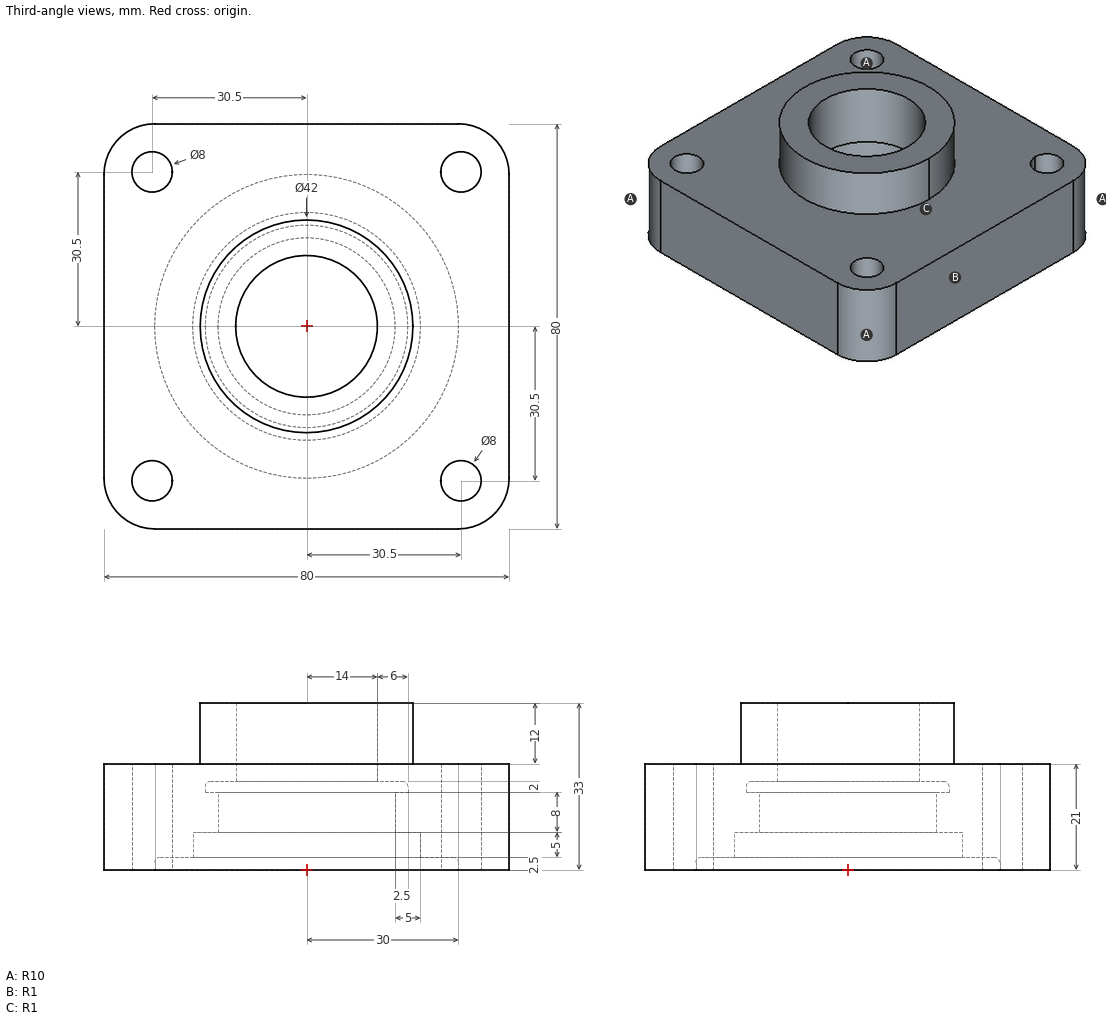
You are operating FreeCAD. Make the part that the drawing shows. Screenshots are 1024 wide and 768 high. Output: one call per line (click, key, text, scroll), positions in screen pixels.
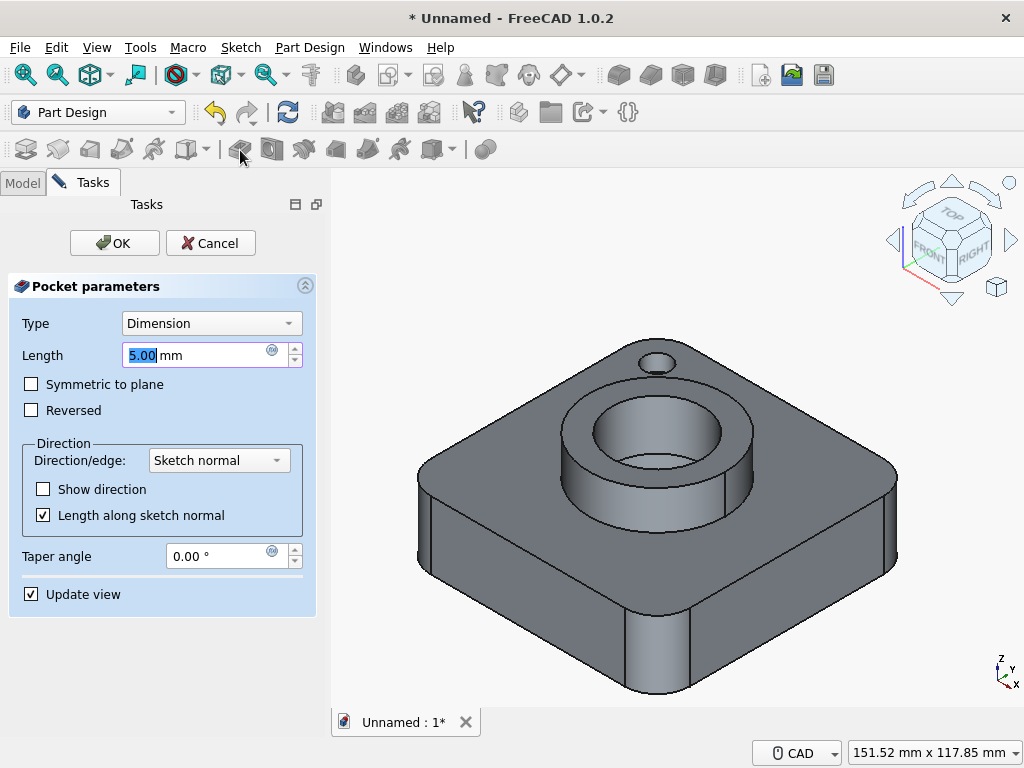
text(21)
key(Tab)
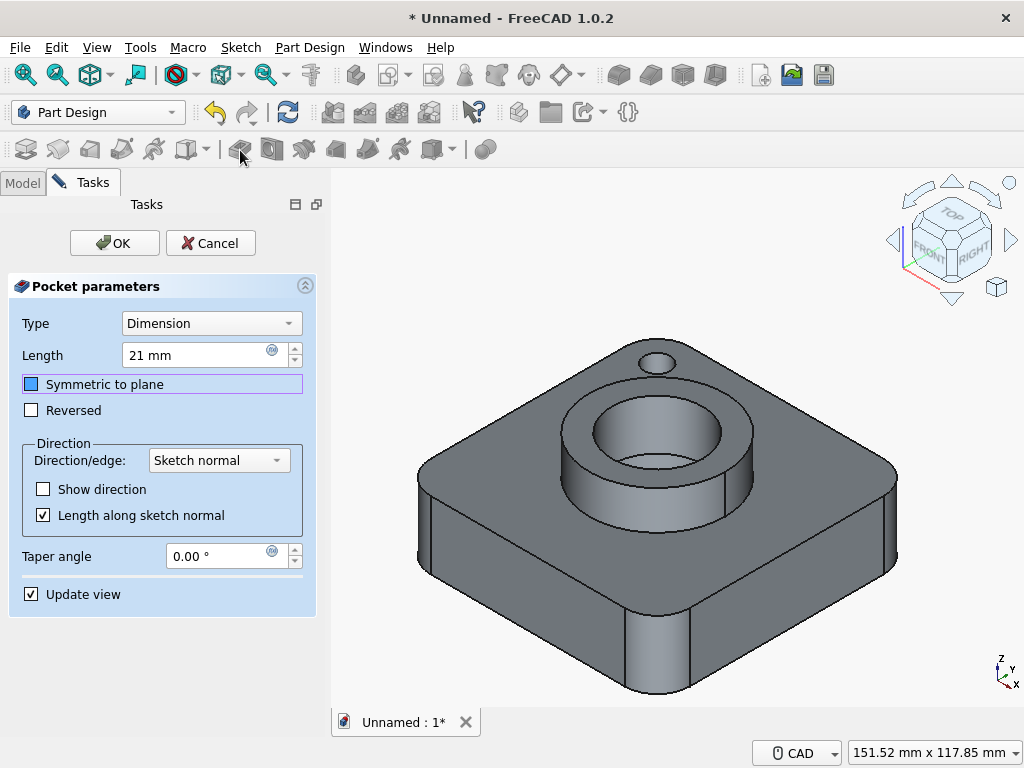
click(115, 243)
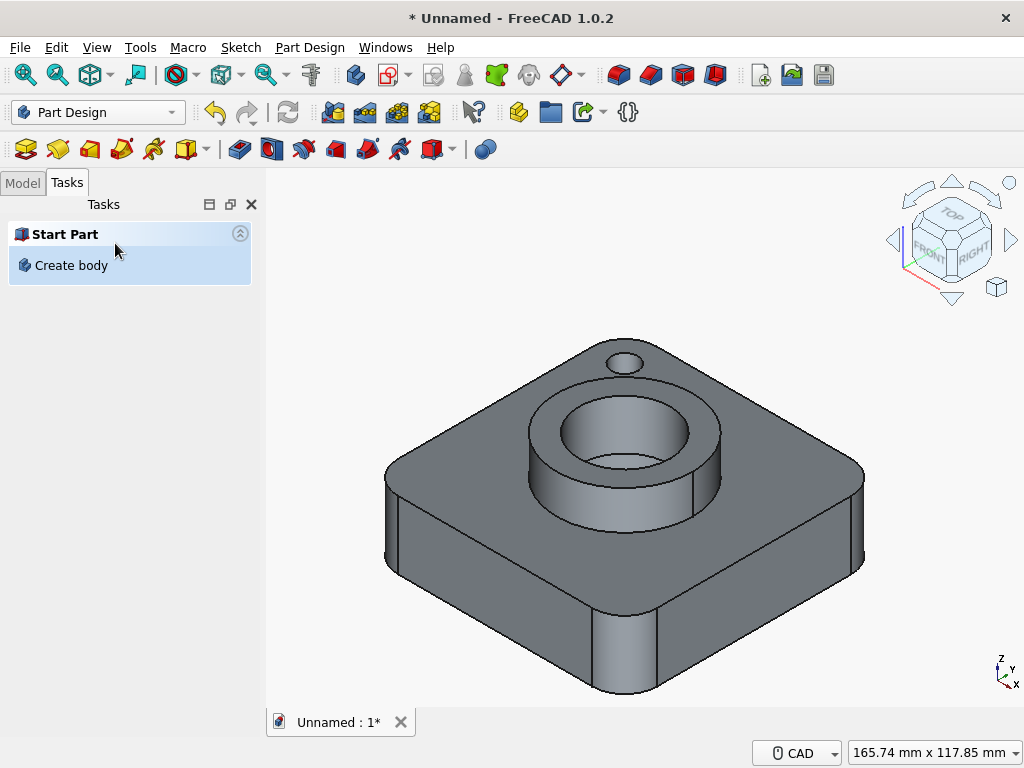
click(23, 182)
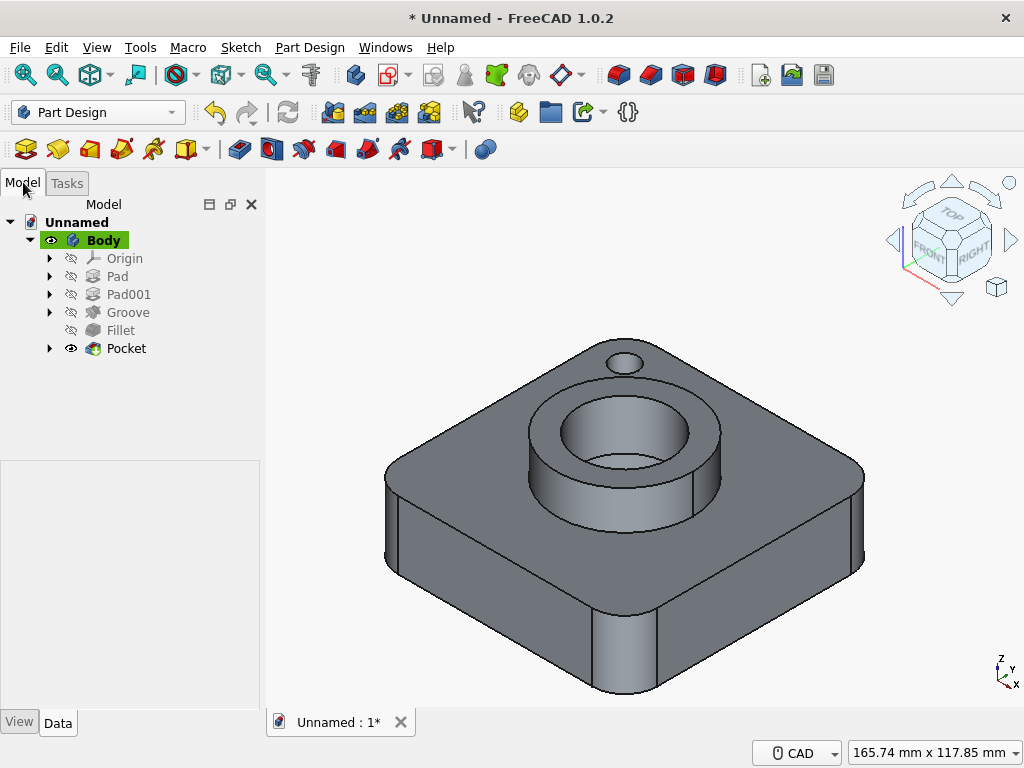
click(116, 348)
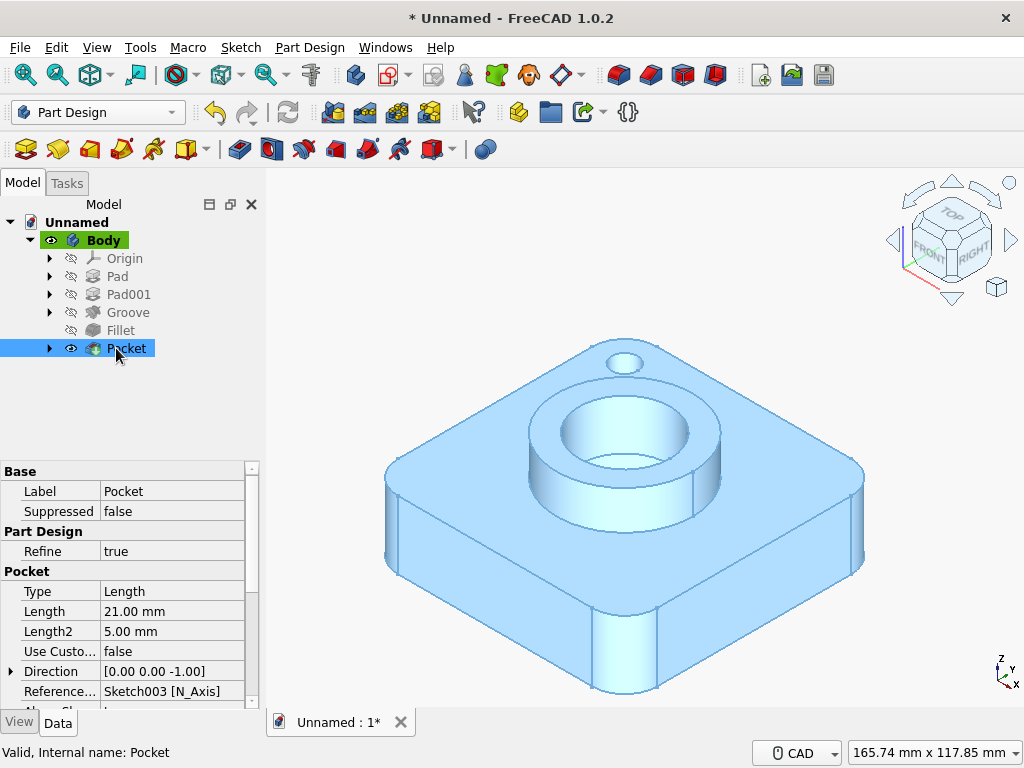
click(334, 112)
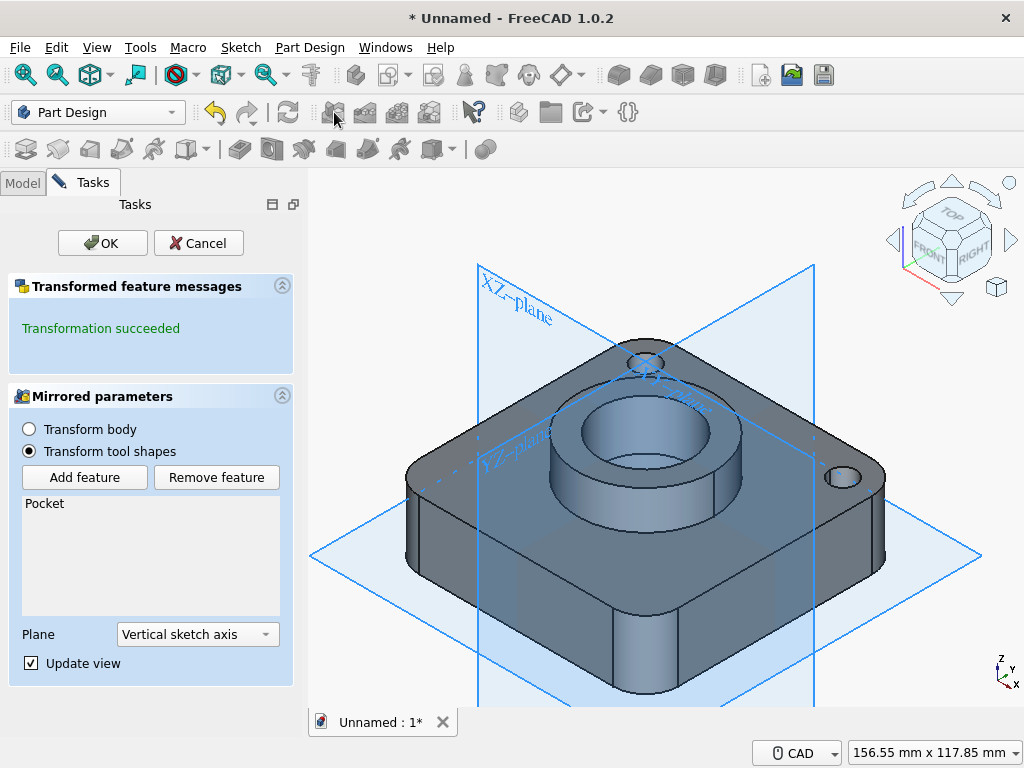
click(198, 634)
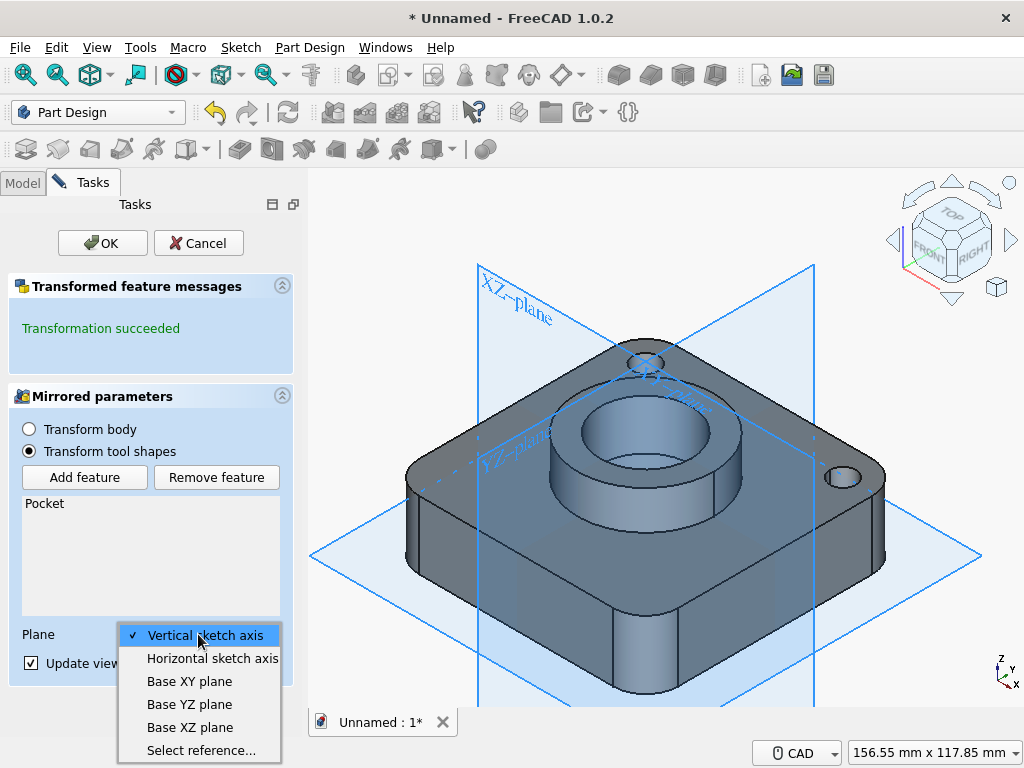
click(198, 728)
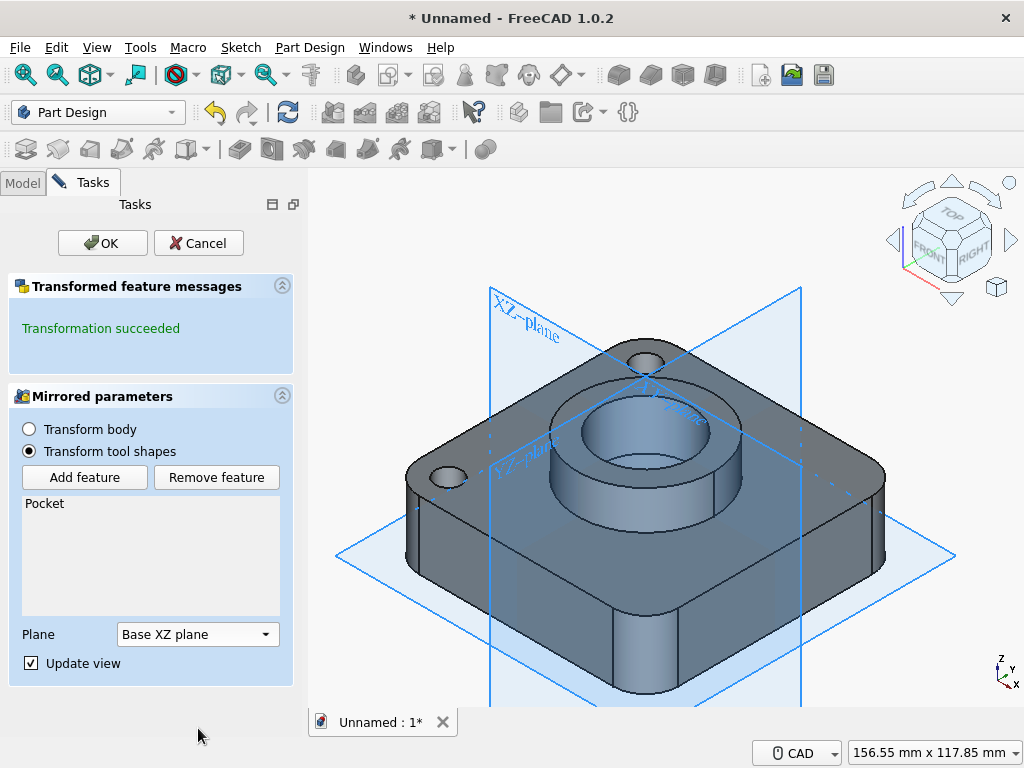
click(103, 243)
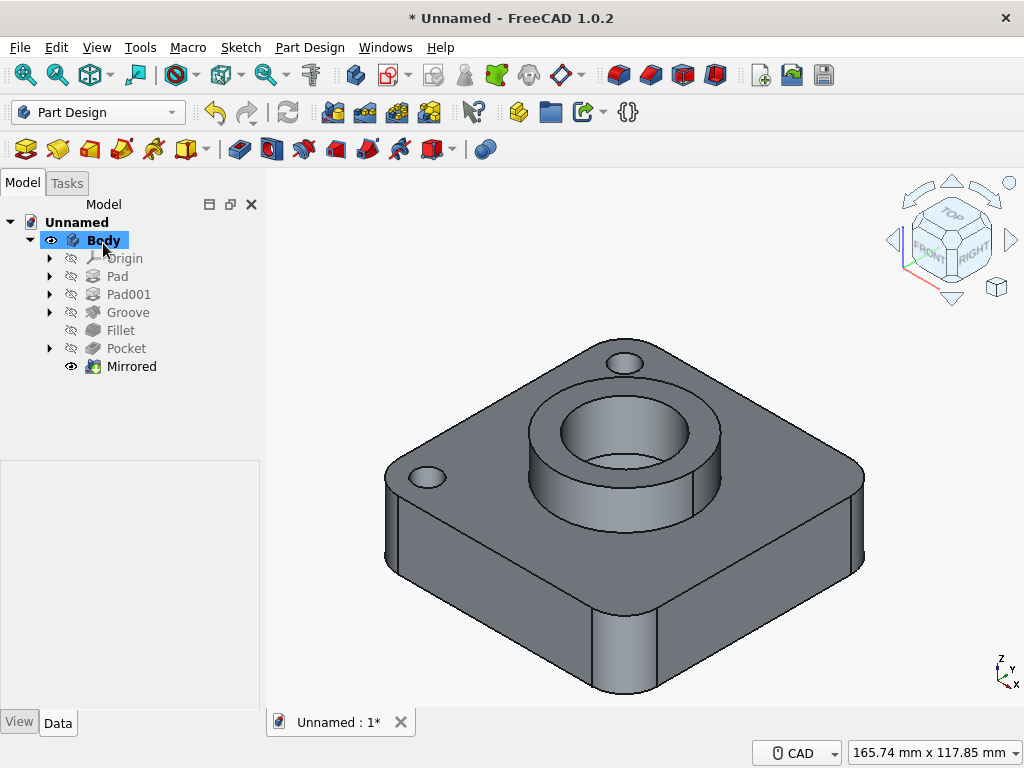
click(116, 348)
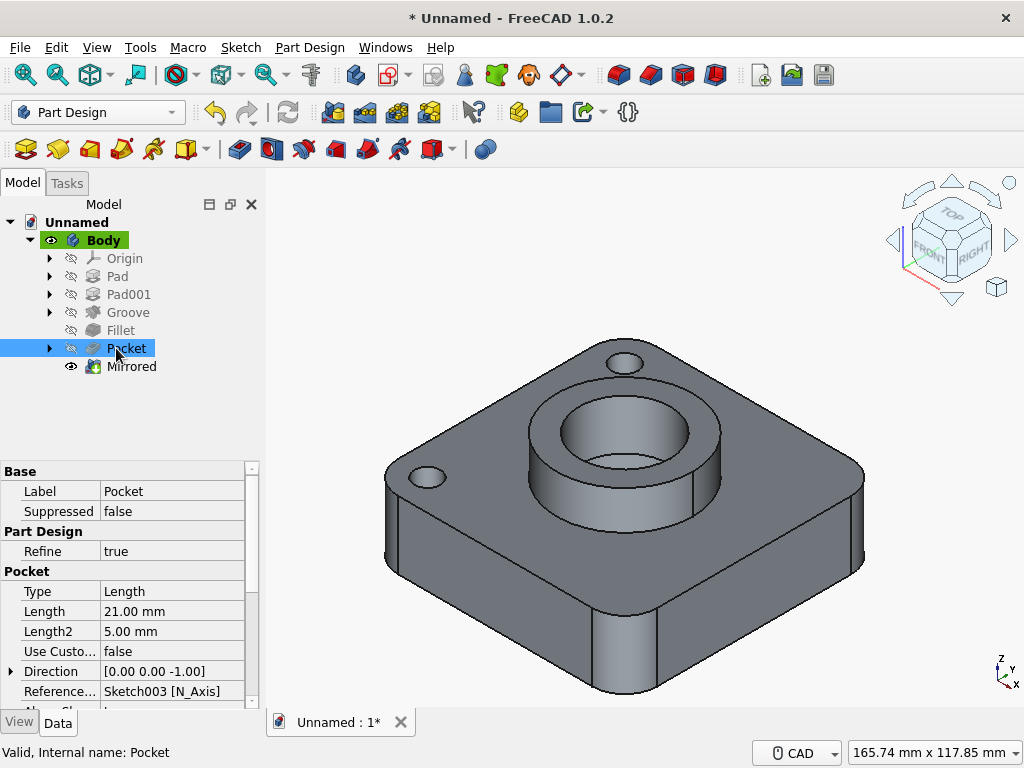
click(334, 112)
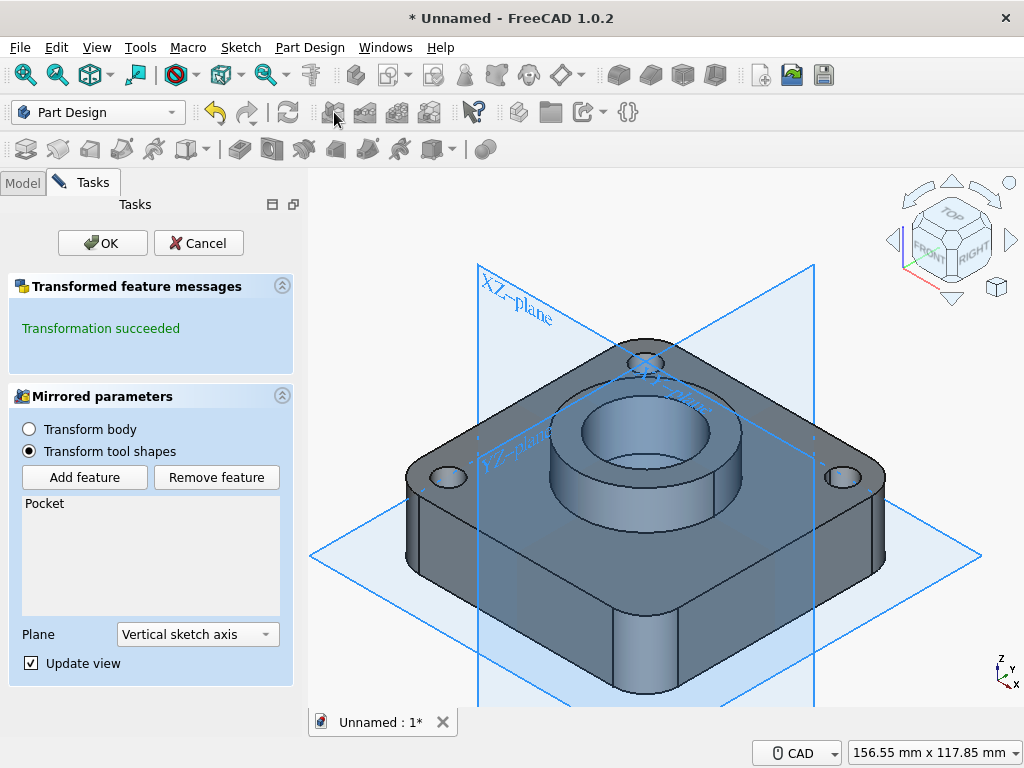
click(198, 634)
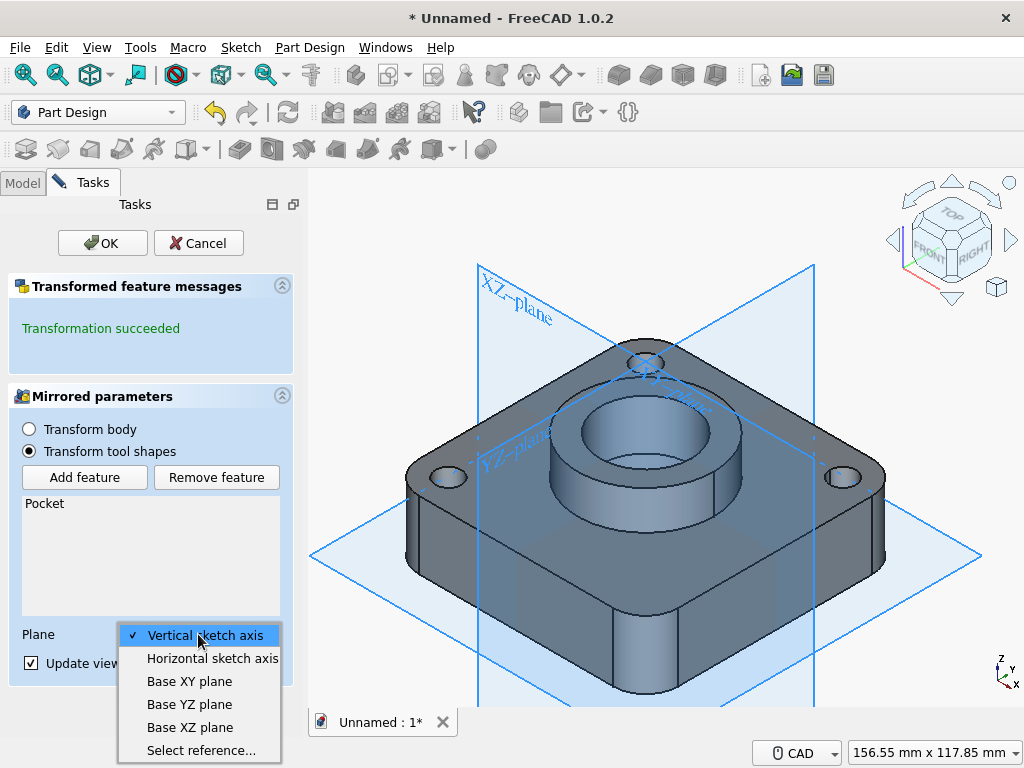
click(198, 704)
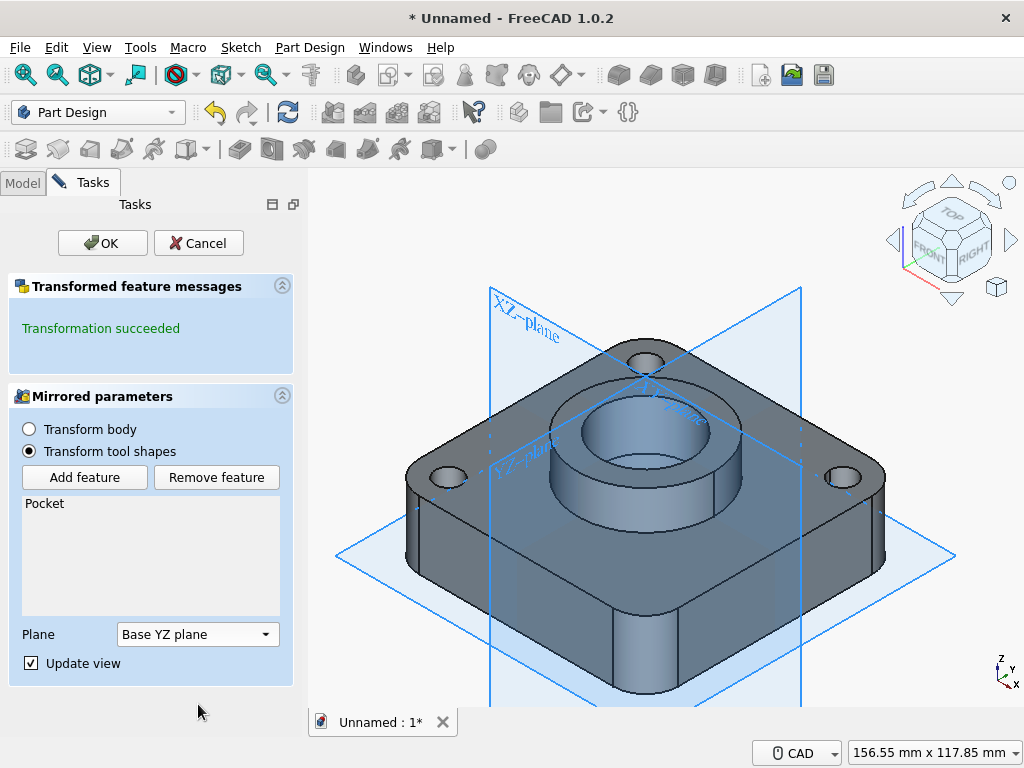
click(103, 243)